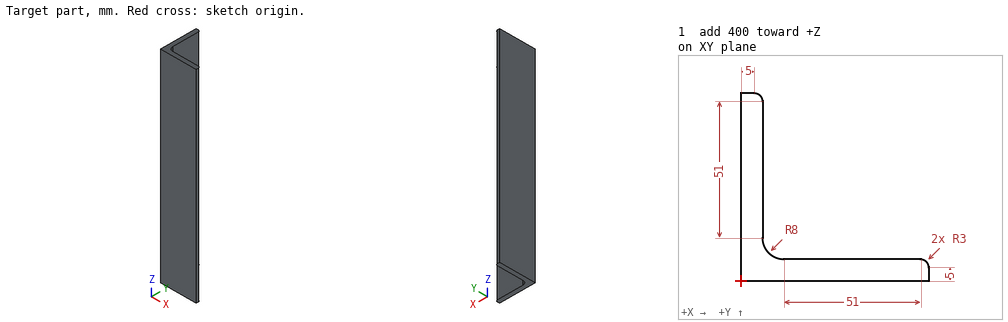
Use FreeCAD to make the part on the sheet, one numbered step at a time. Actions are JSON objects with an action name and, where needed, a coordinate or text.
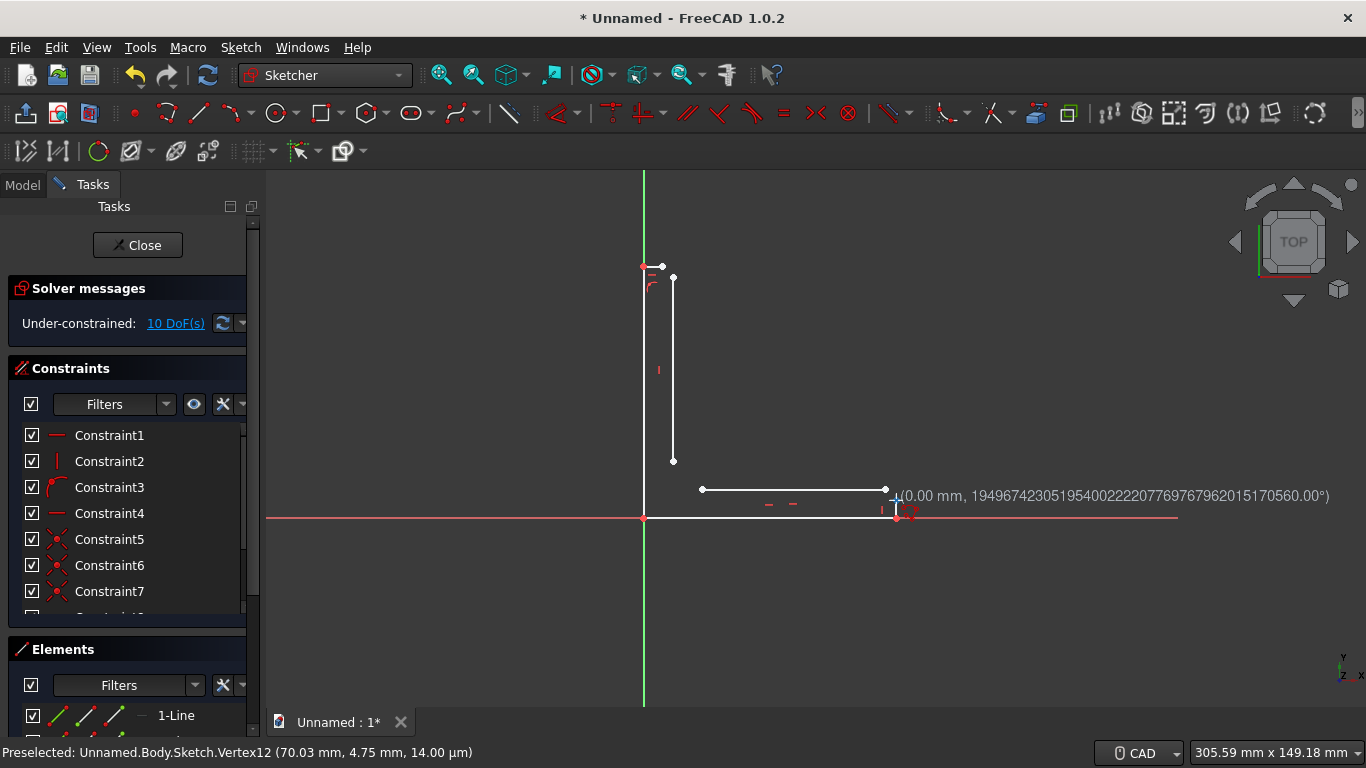
{"action": "left_click", "coordinate": [232, 114]}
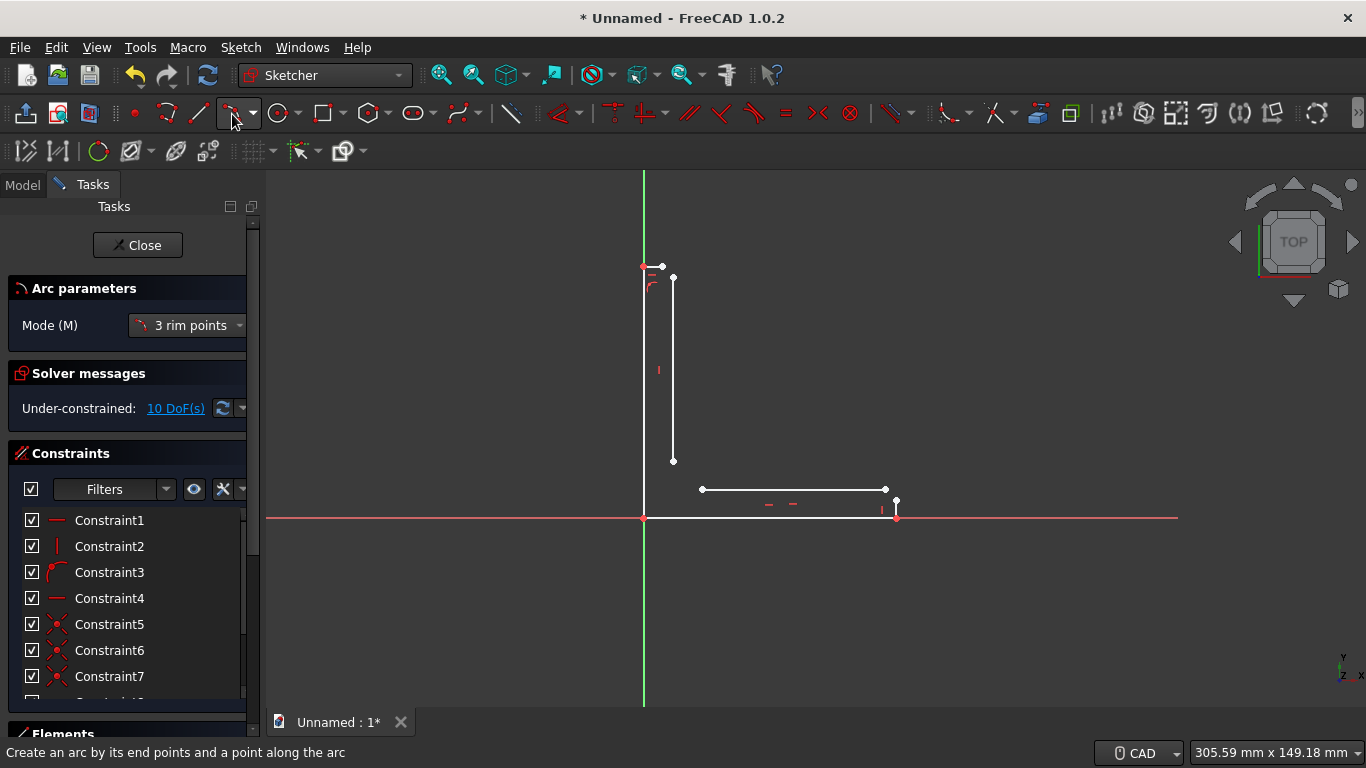
{"action": "left_click", "coordinate": [702, 490]}
{"action": "left_click", "coordinate": [673, 462]}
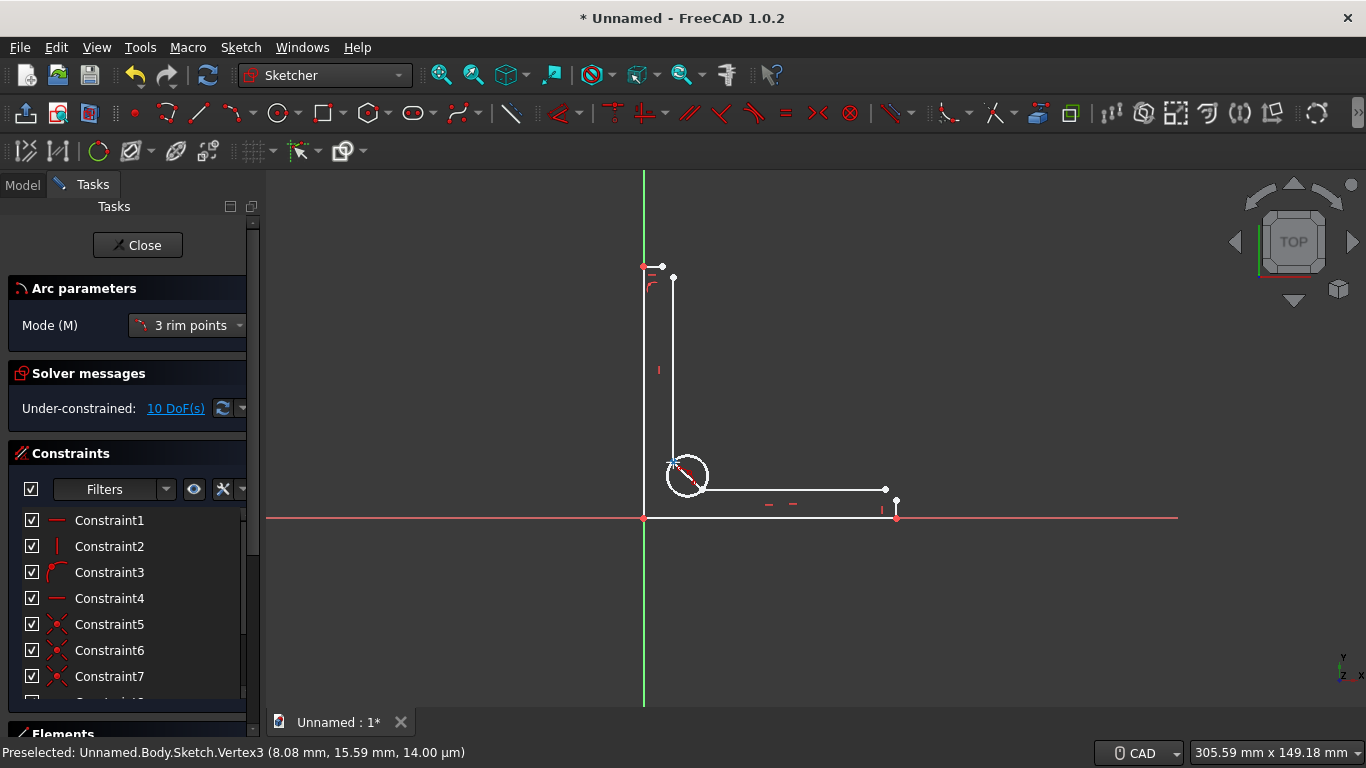
{"action": "scroll", "coordinate": [681, 481], "scroll_direction": "up", "scroll_amount": 4}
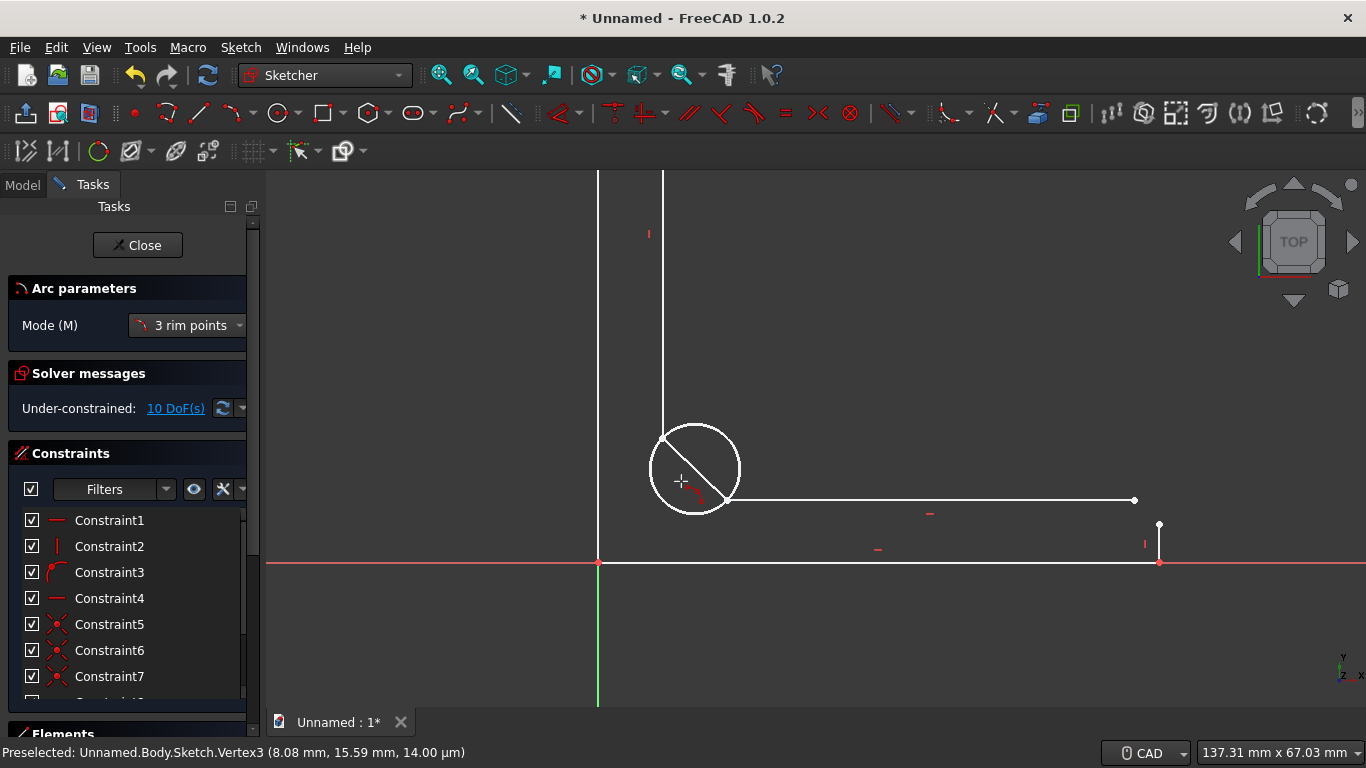
{"action": "left_click", "coordinate": [681, 480]}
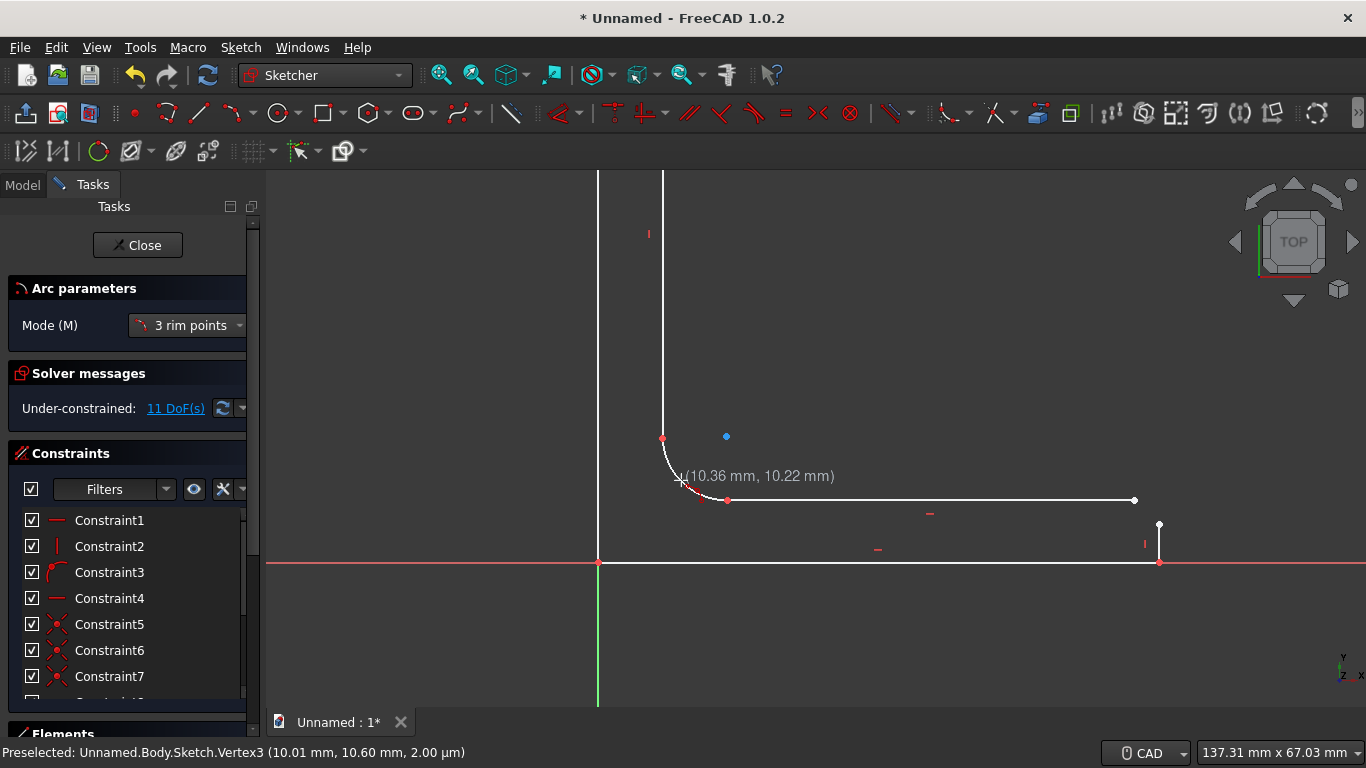
{"action": "scroll", "coordinate": [588, 628], "scroll_direction": "down", "scroll_amount": 3}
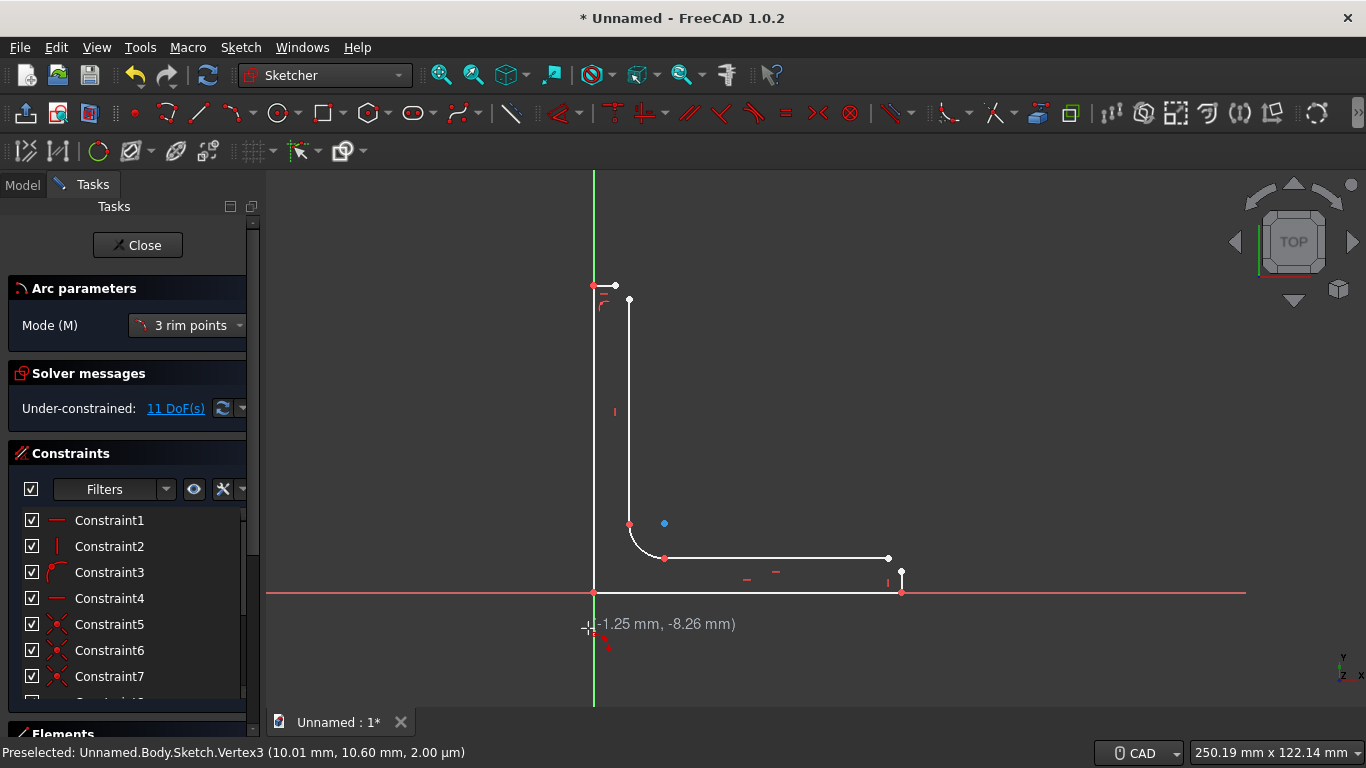
{"action": "left_click", "coordinate": [629, 299]}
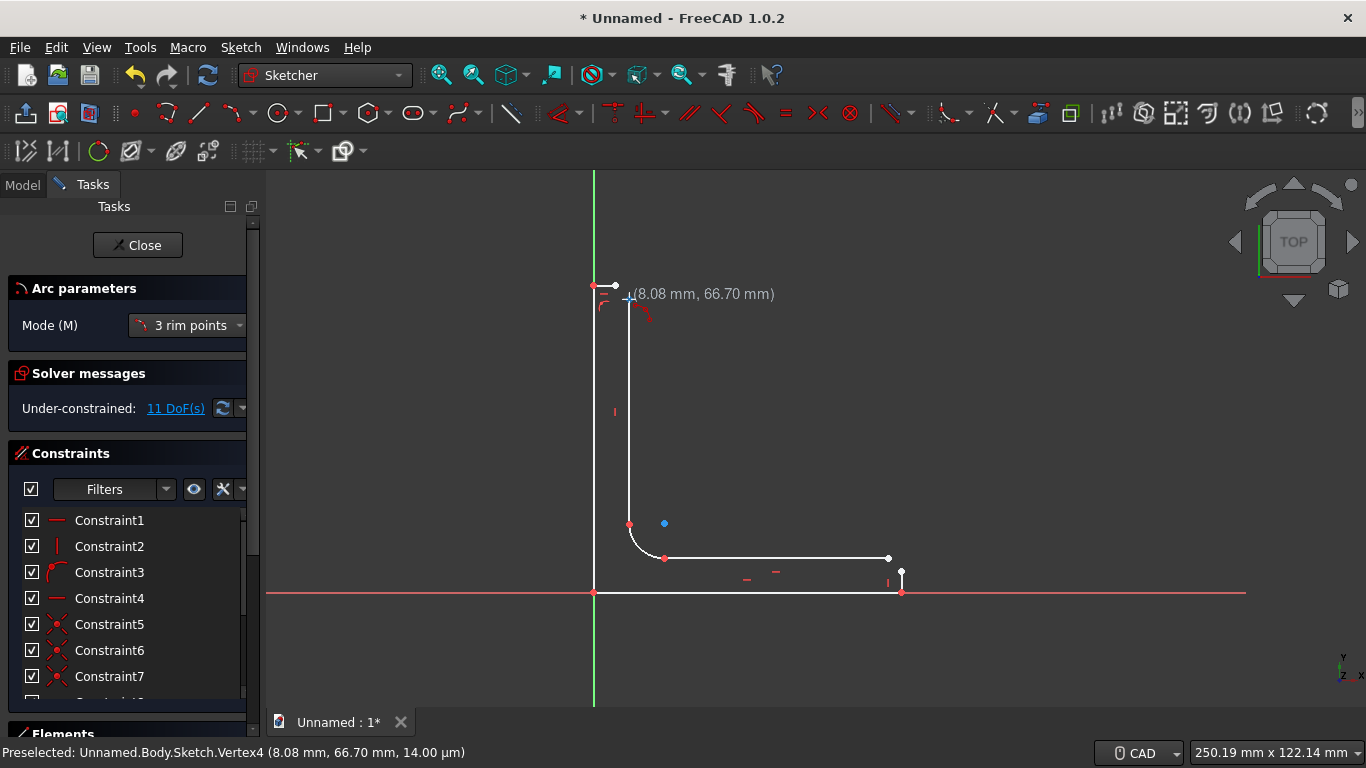
{"action": "scroll", "coordinate": [616, 285], "scroll_direction": "up", "scroll_amount": 2}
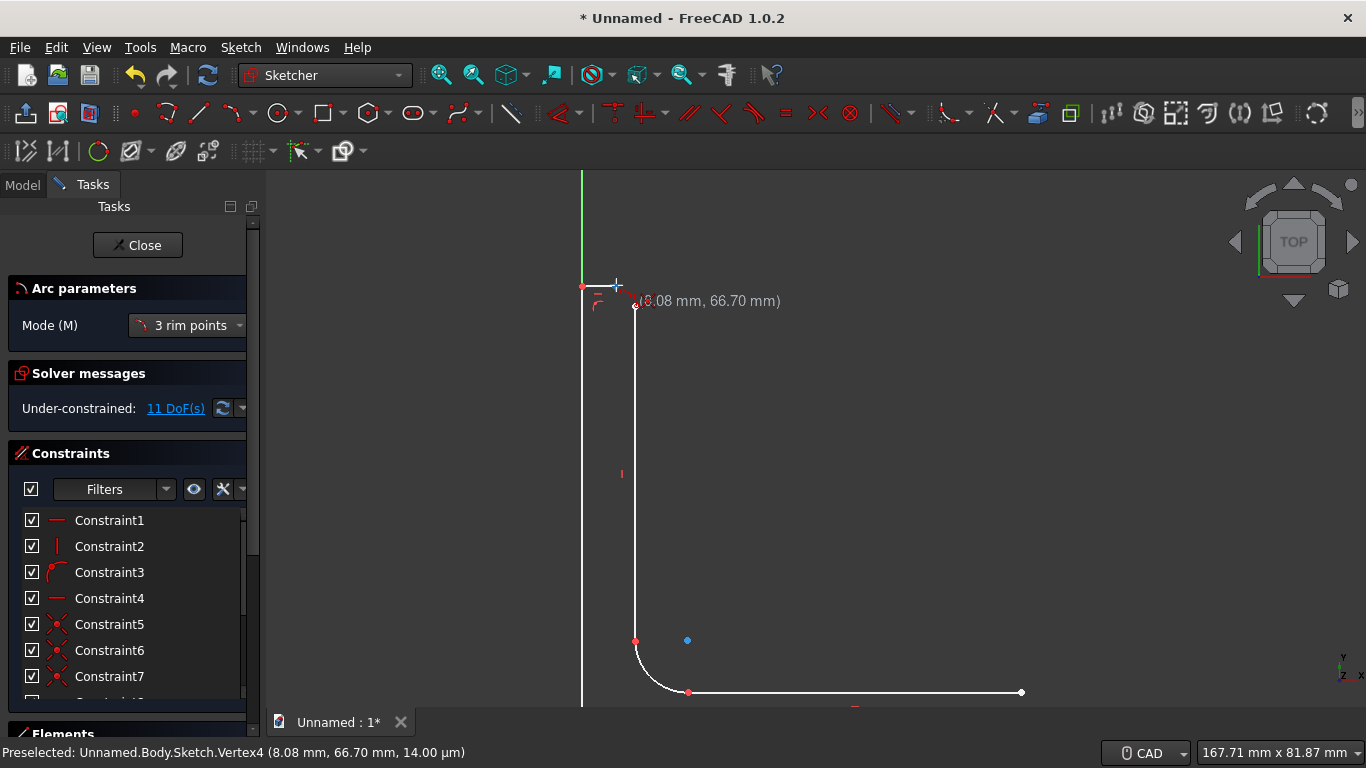
{"action": "left_click", "coordinate": [615, 286]}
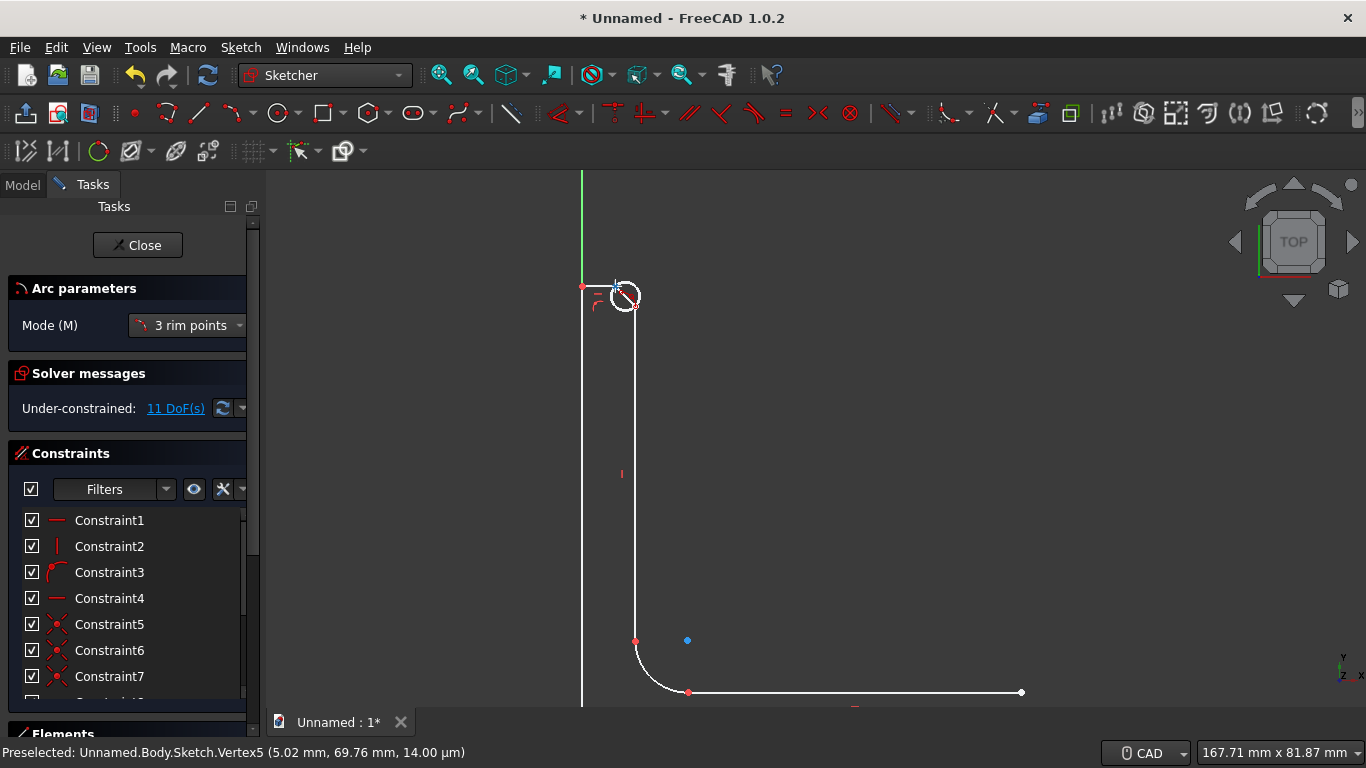
{"action": "scroll", "coordinate": [629, 290], "scroll_direction": "up", "scroll_amount": 6}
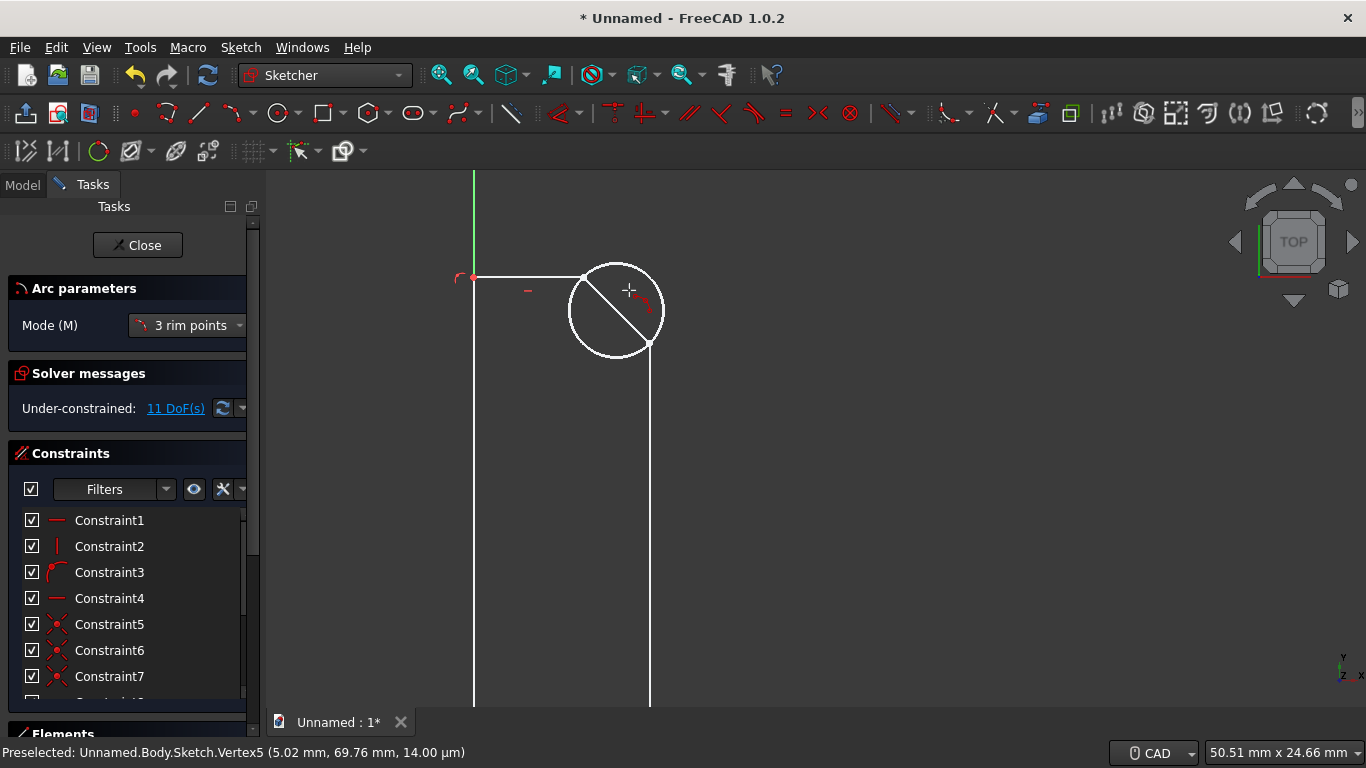
{"action": "left_click", "coordinate": [629, 291]}